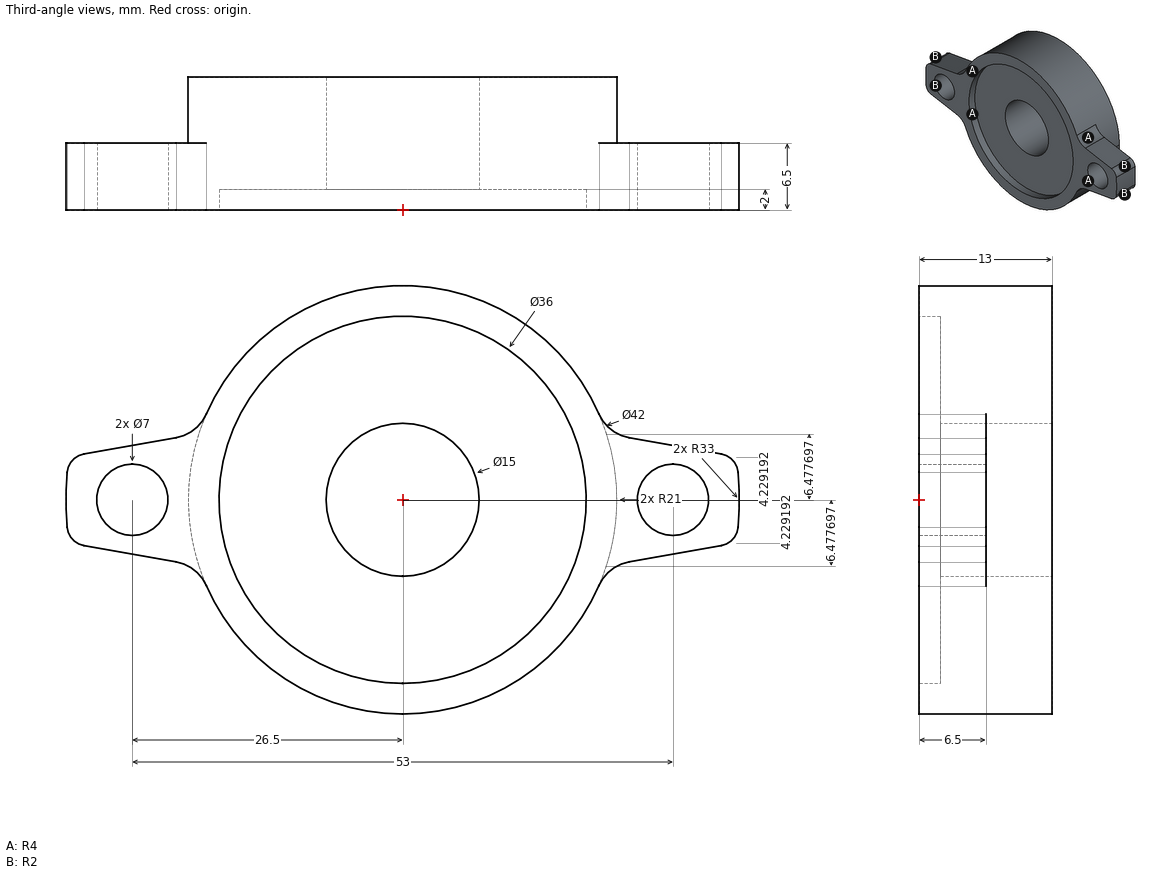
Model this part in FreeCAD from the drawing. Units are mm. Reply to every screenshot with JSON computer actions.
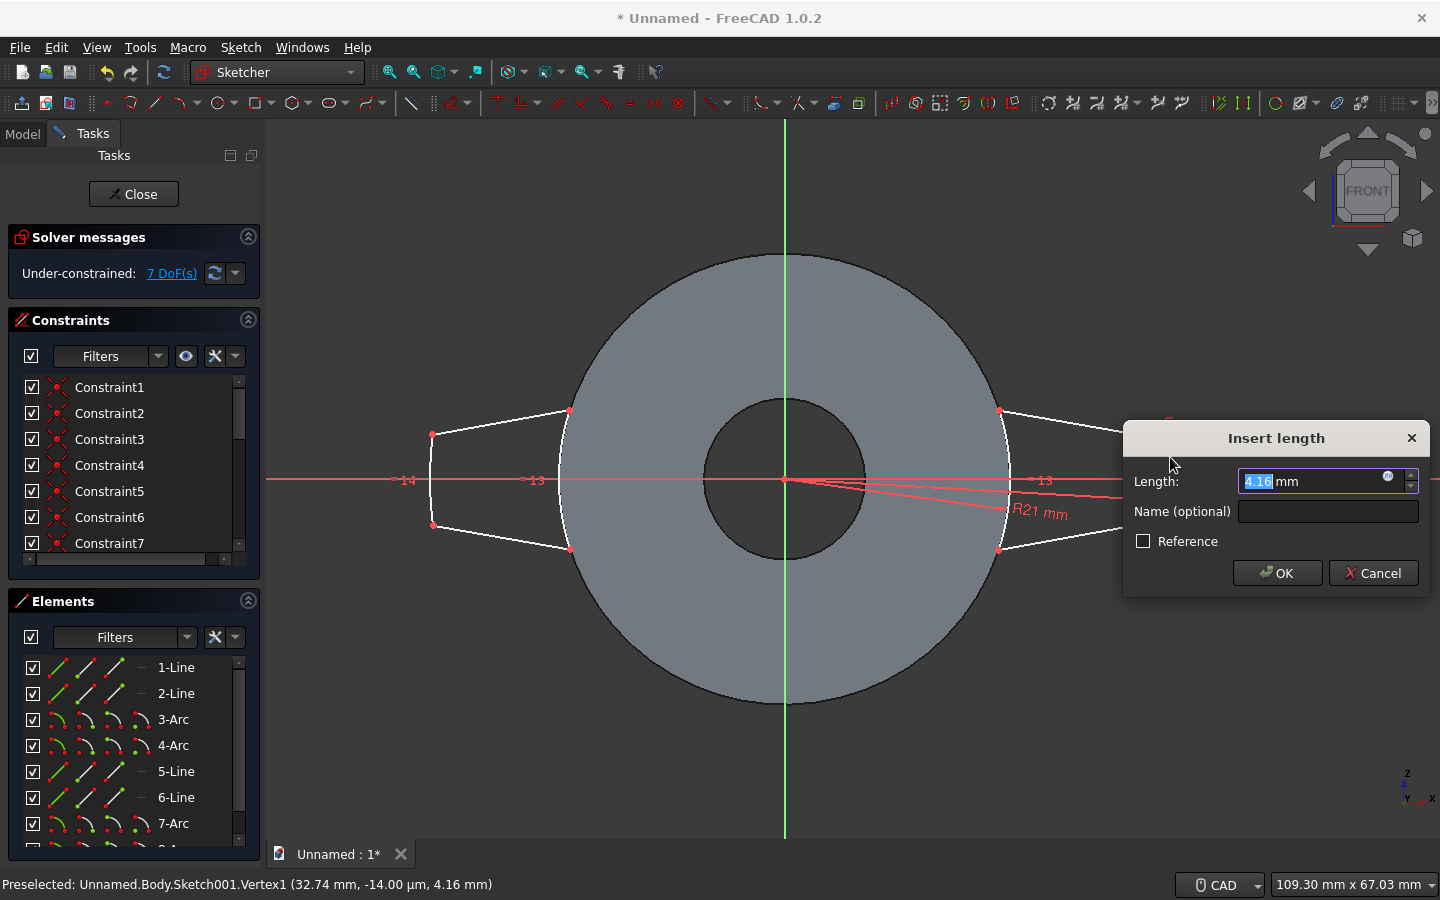
{"action": "type", "text": "4.229192"}
{"action": "key", "text": "Return"}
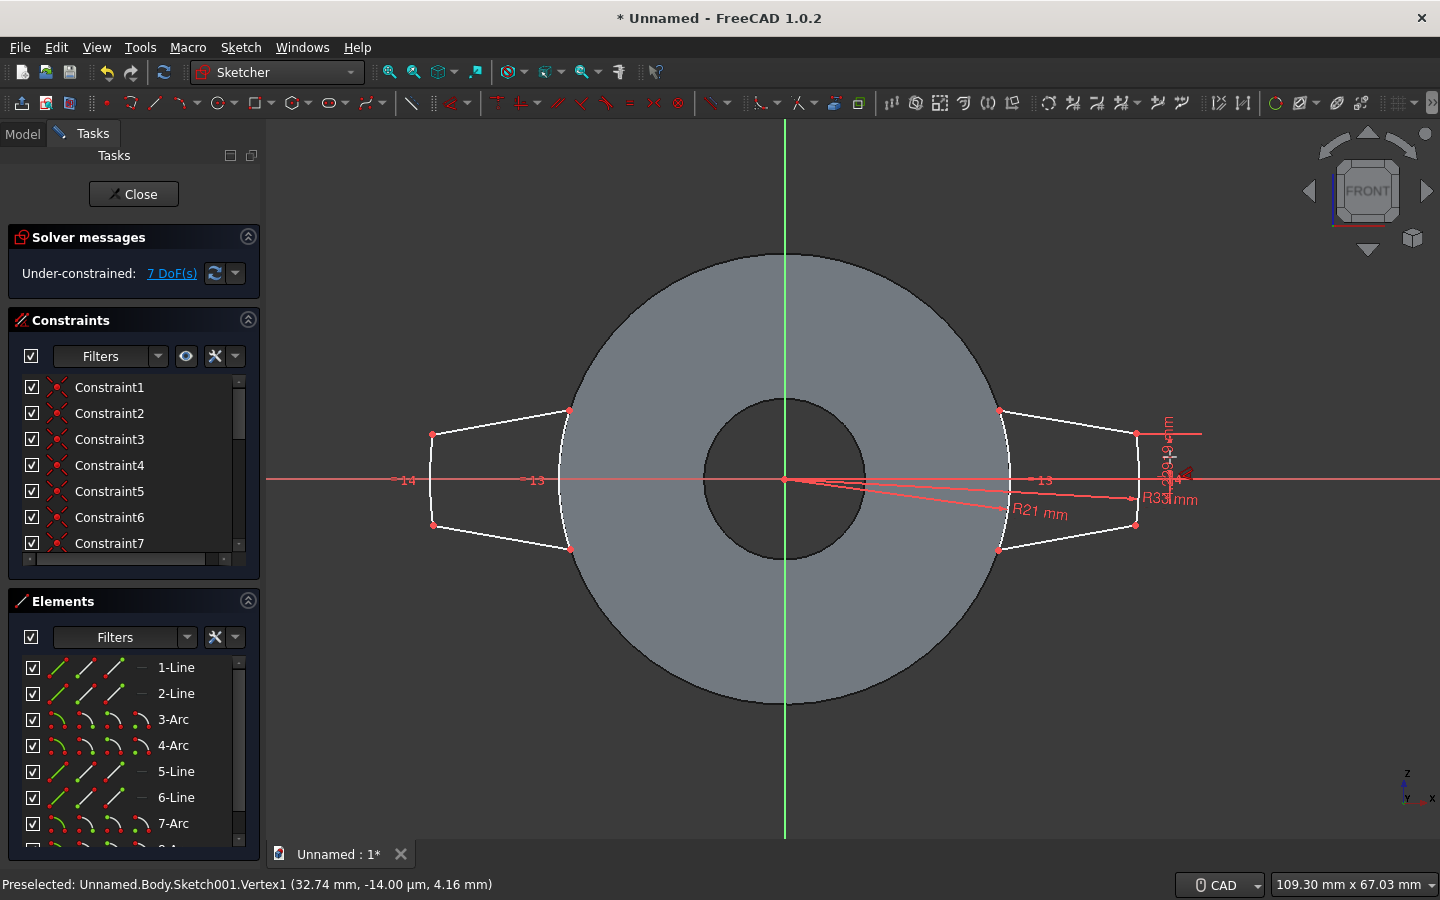
{"action": "left_click", "coordinate": [999, 411]}
{"action": "left_click", "coordinate": [1033, 445]}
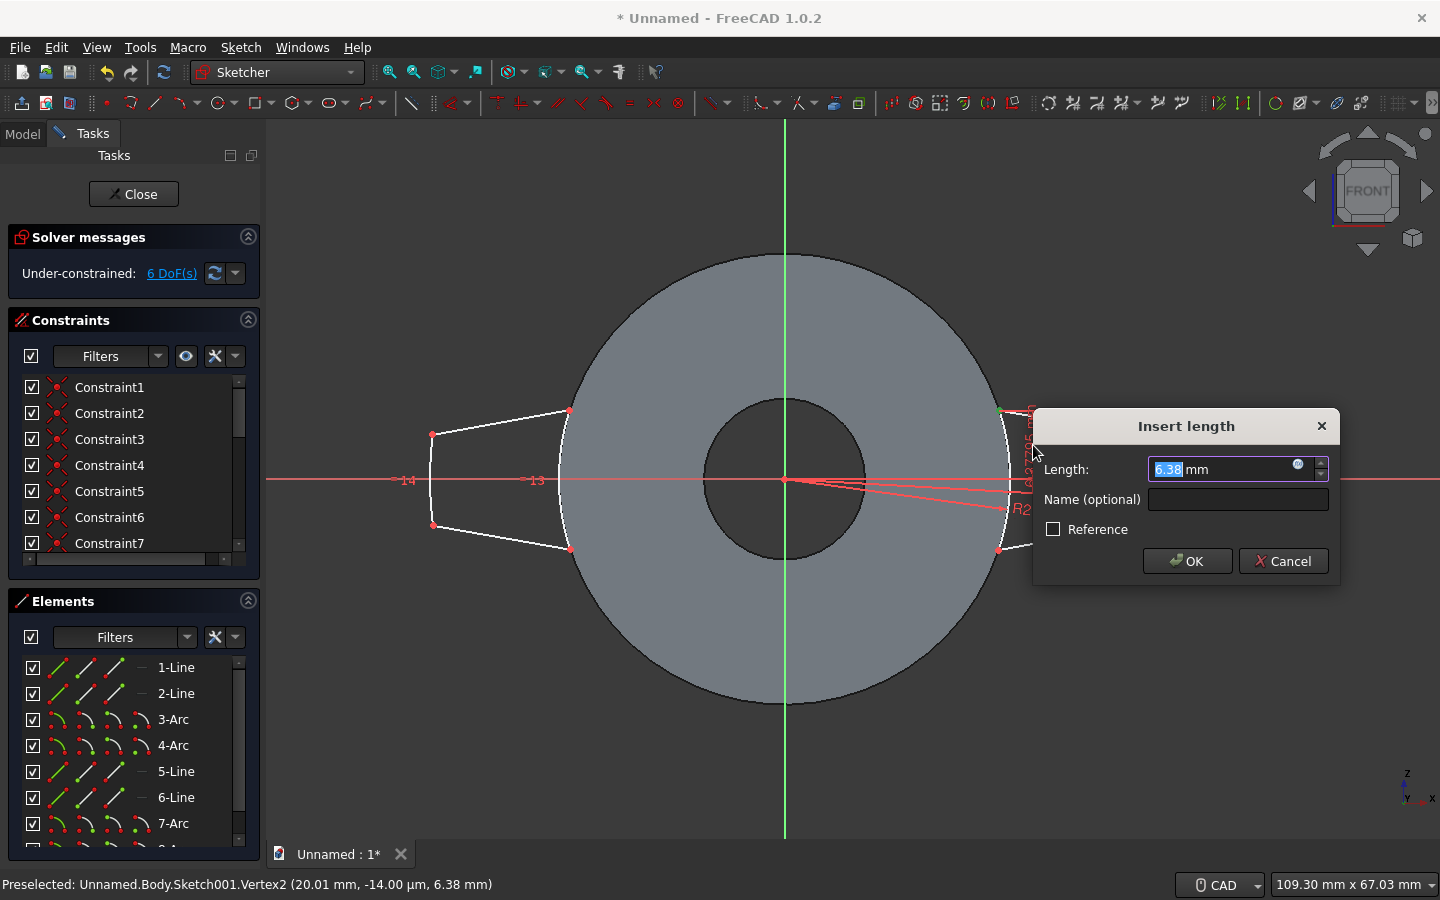
{"action": "type", "text": "6.477697"}
{"action": "key", "text": "Return"}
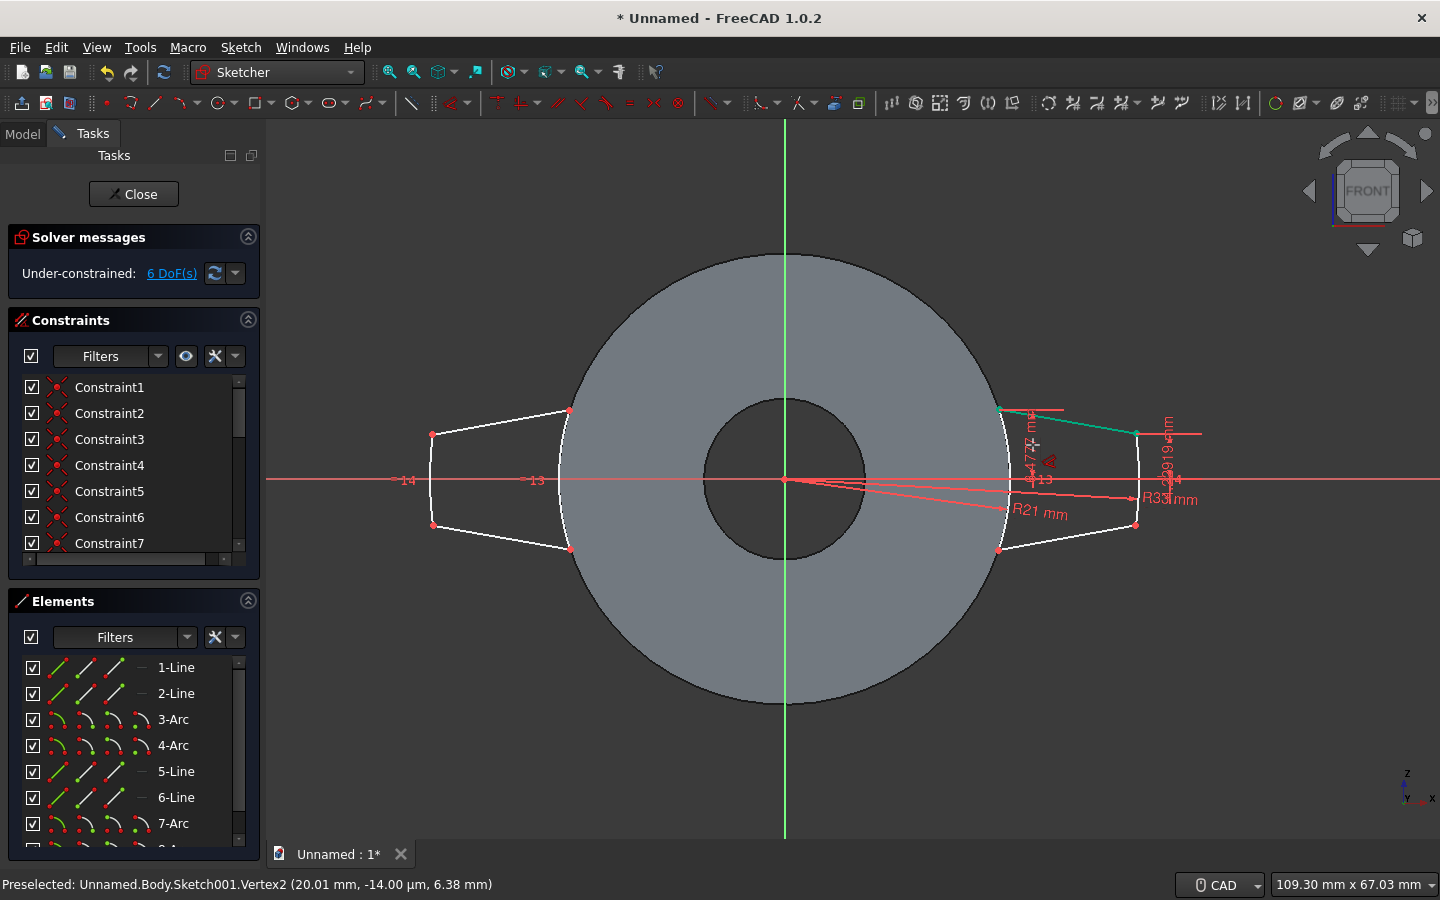
{"action": "left_click", "coordinate": [999, 550]}
{"action": "left_click", "coordinate": [751, 515]}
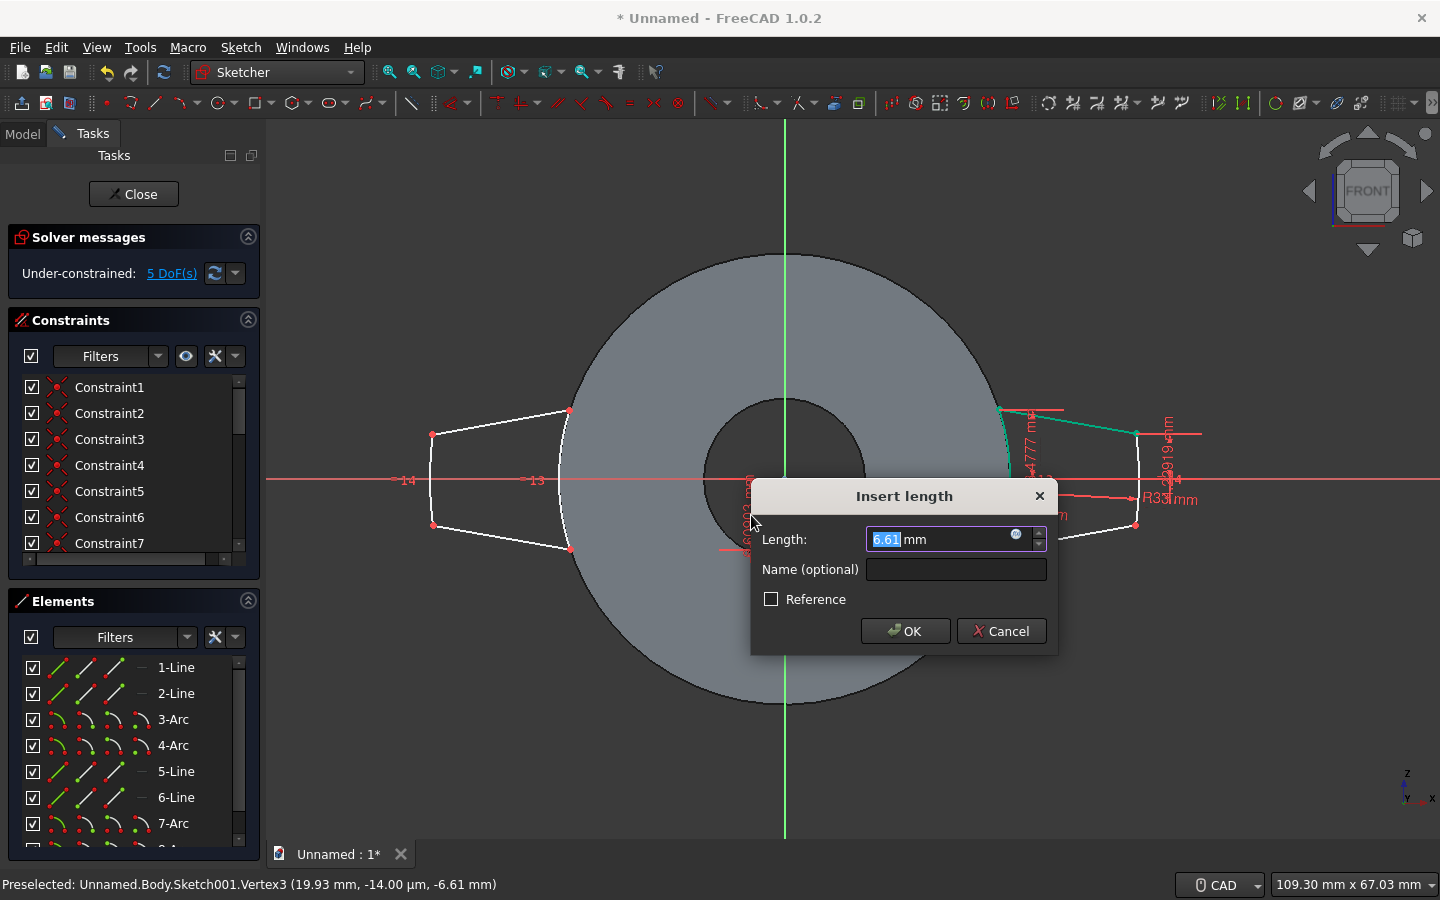
{"action": "type", "text": "6.477697"}
{"action": "key", "text": "Return"}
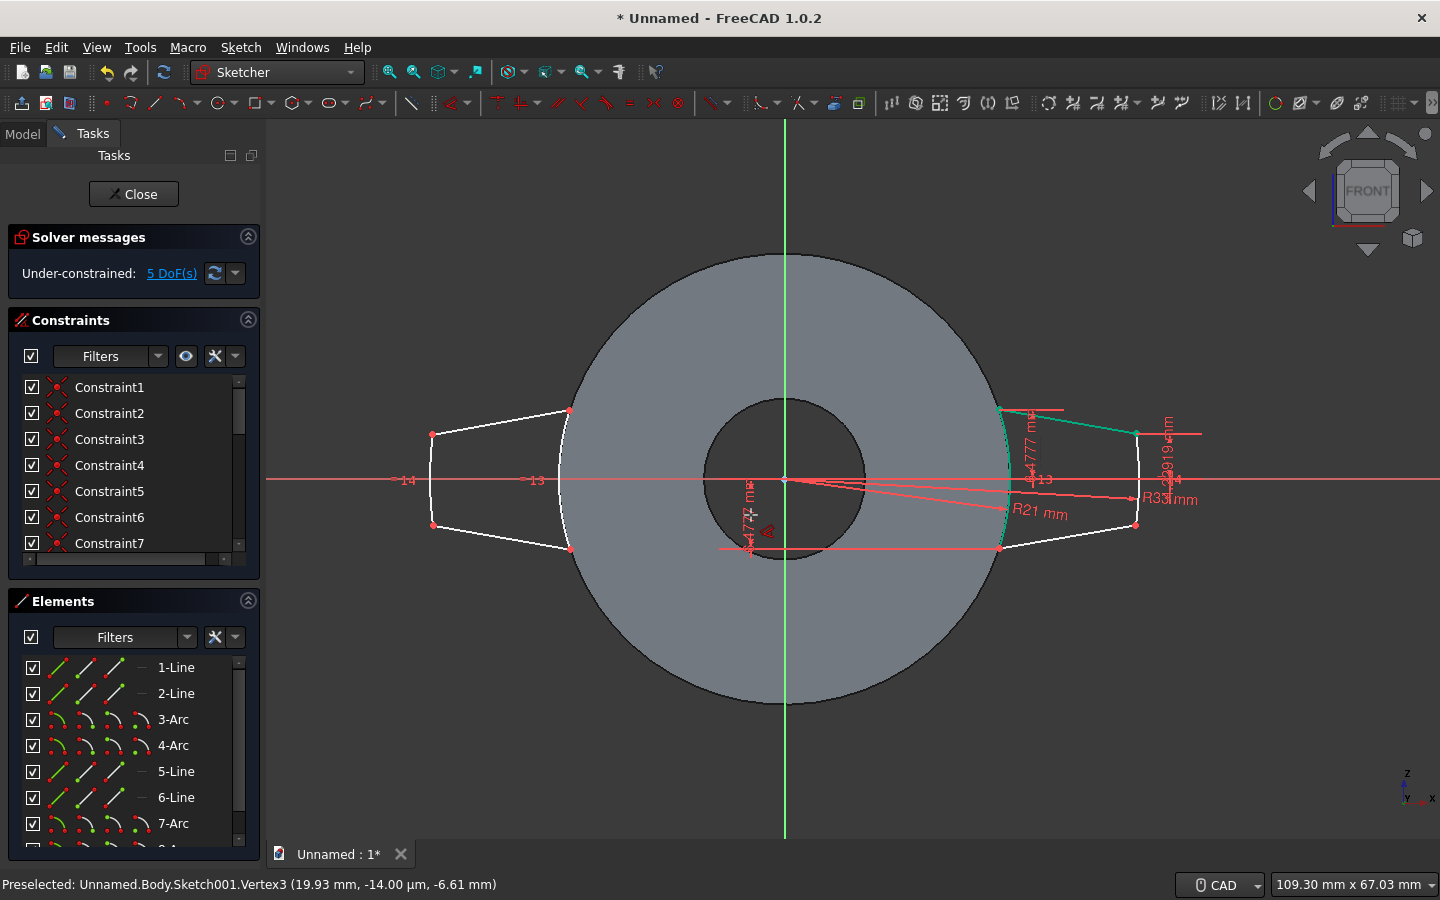
{"action": "left_click", "coordinate": [1136, 525]}
{"action": "left_click", "coordinate": [1242, 502]}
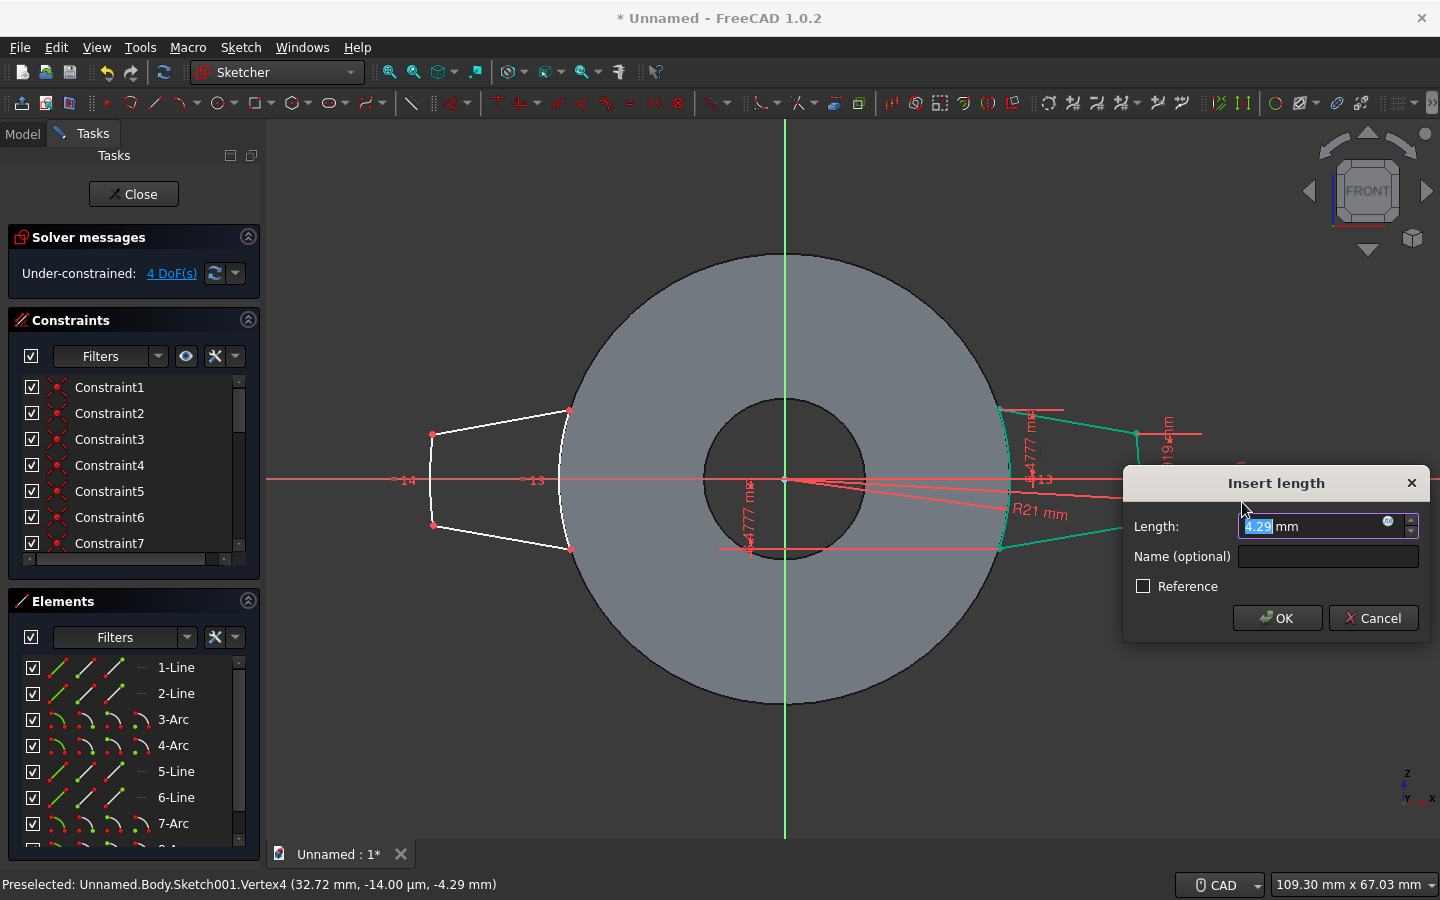
{"action": "type", "text": "4.229192"}
{"action": "key", "text": "Return"}